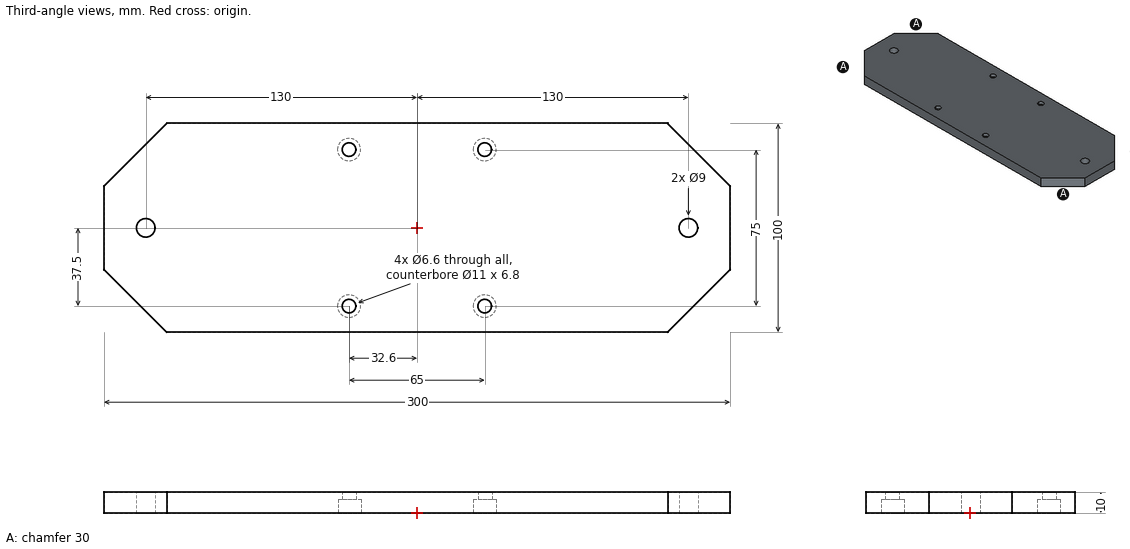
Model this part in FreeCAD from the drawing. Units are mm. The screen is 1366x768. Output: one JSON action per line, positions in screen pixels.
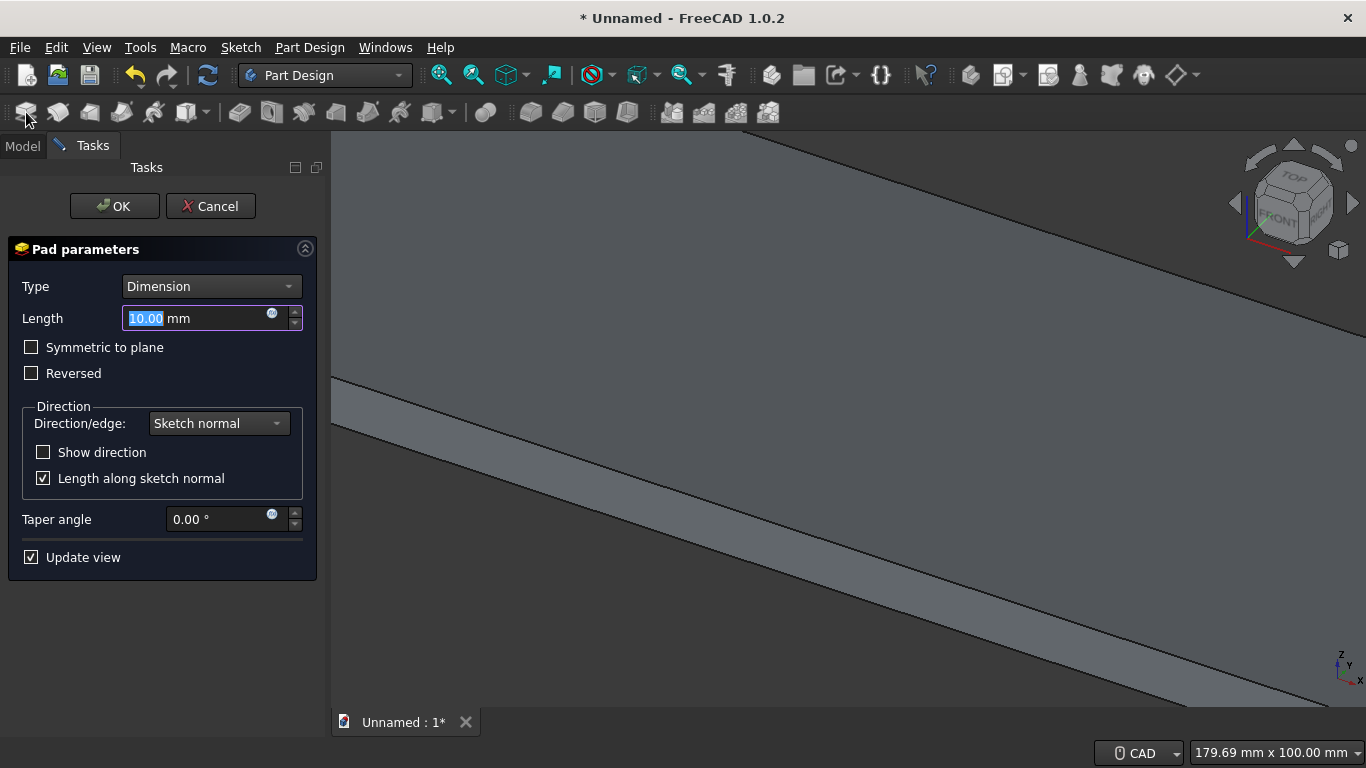
{"action": "type", "text": "10"}
{"action": "key", "text": "Tab"}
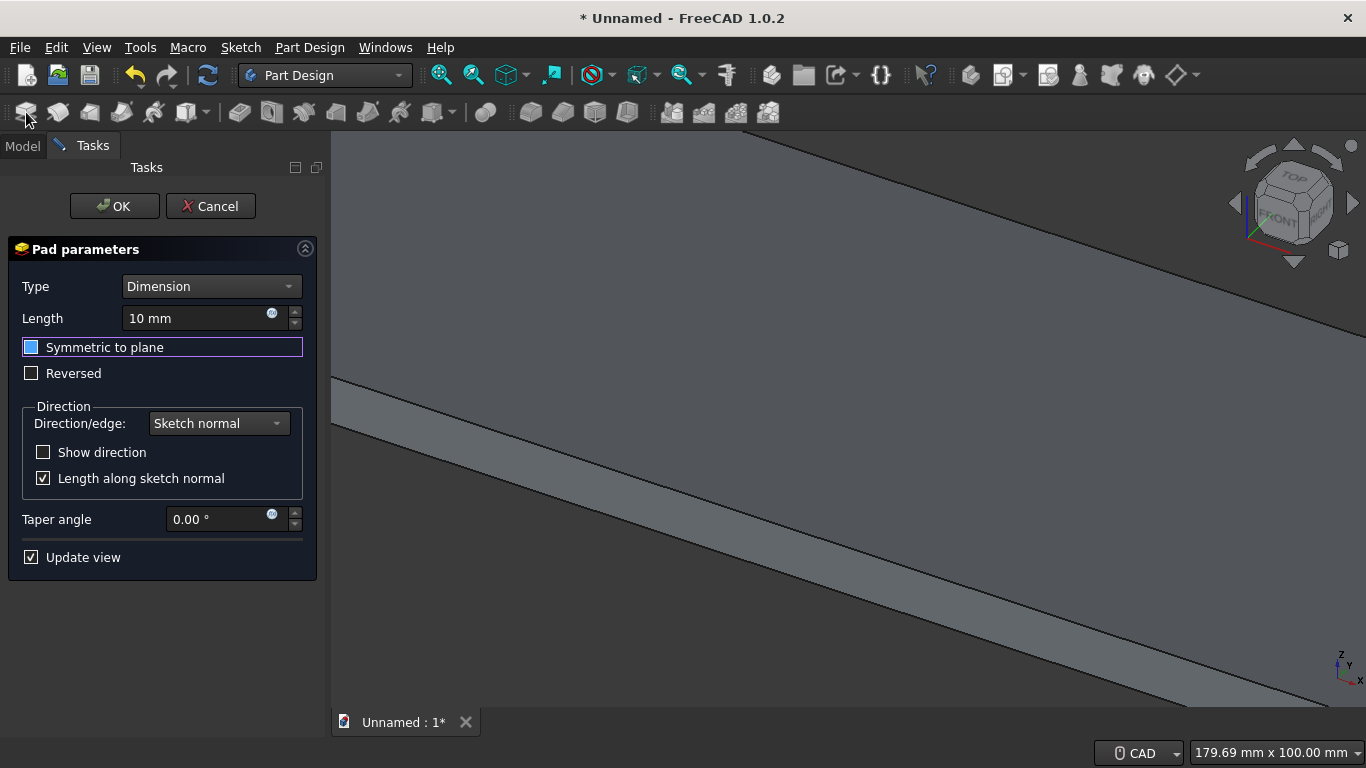
{"action": "left_click", "coordinate": [115, 206]}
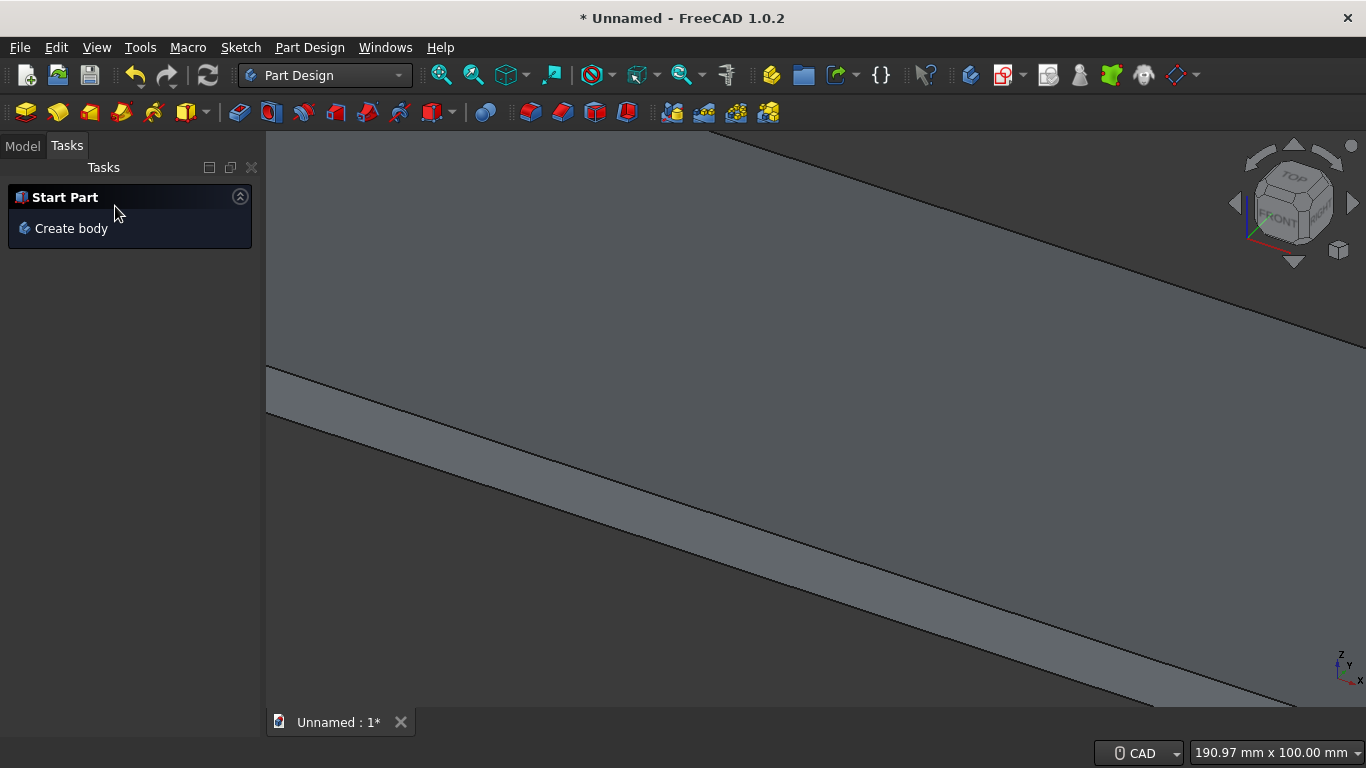
{"action": "key", "text": "v f"}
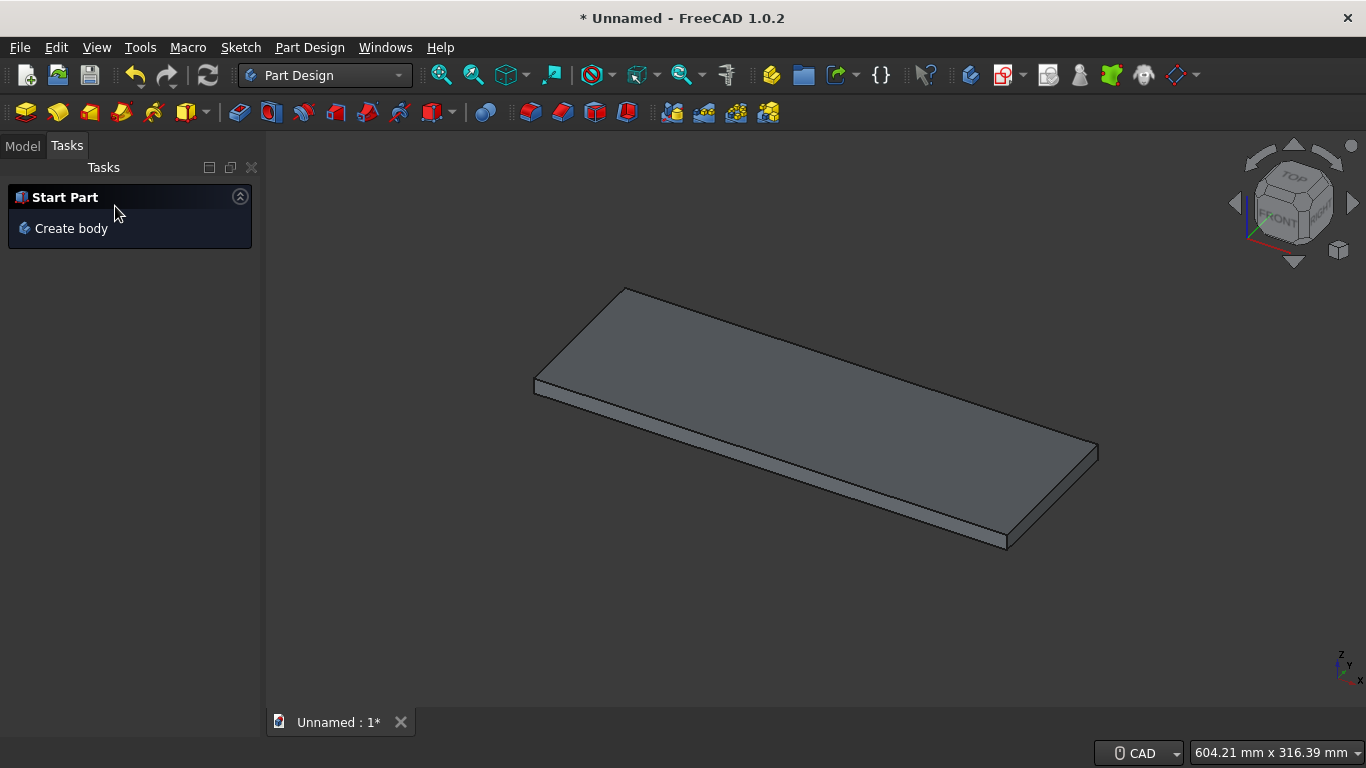
{"action": "key", "text": "5"}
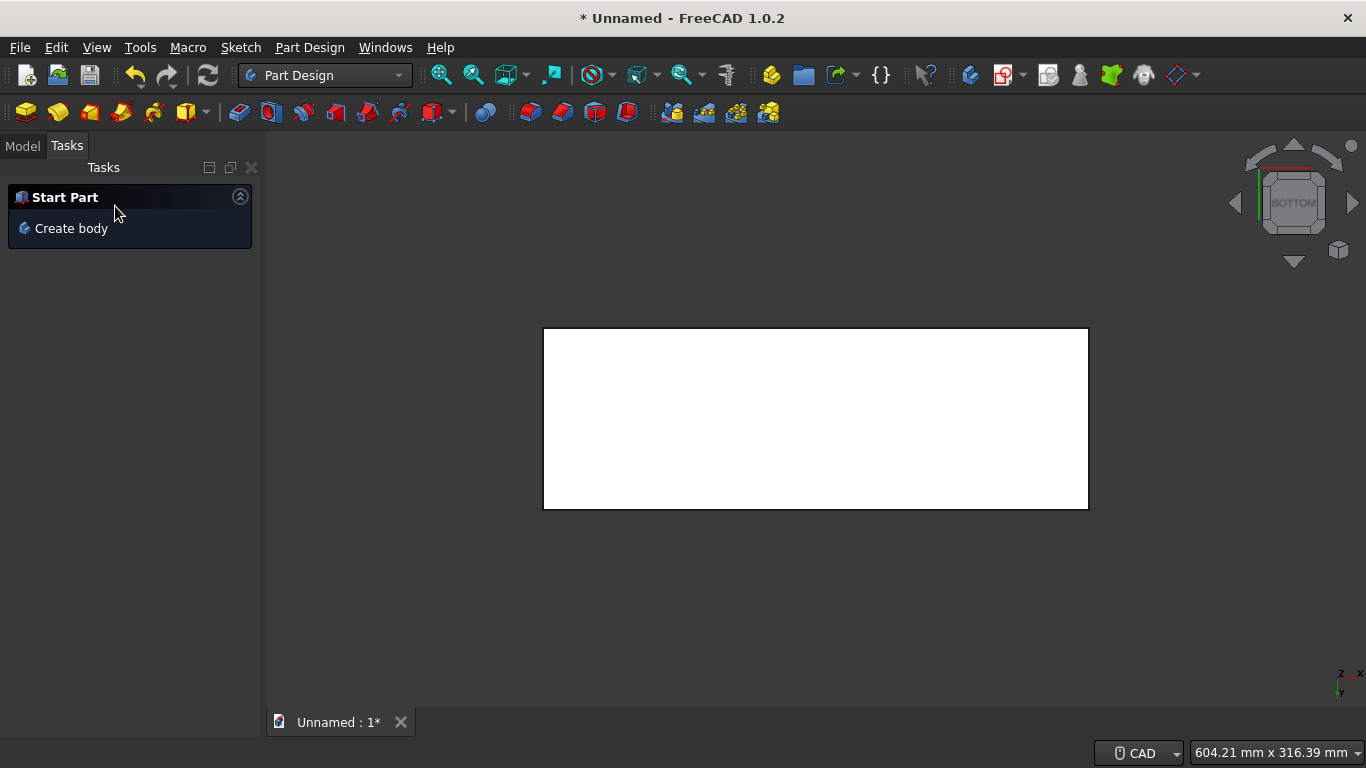
{"action": "left_click", "coordinate": [972, 418]}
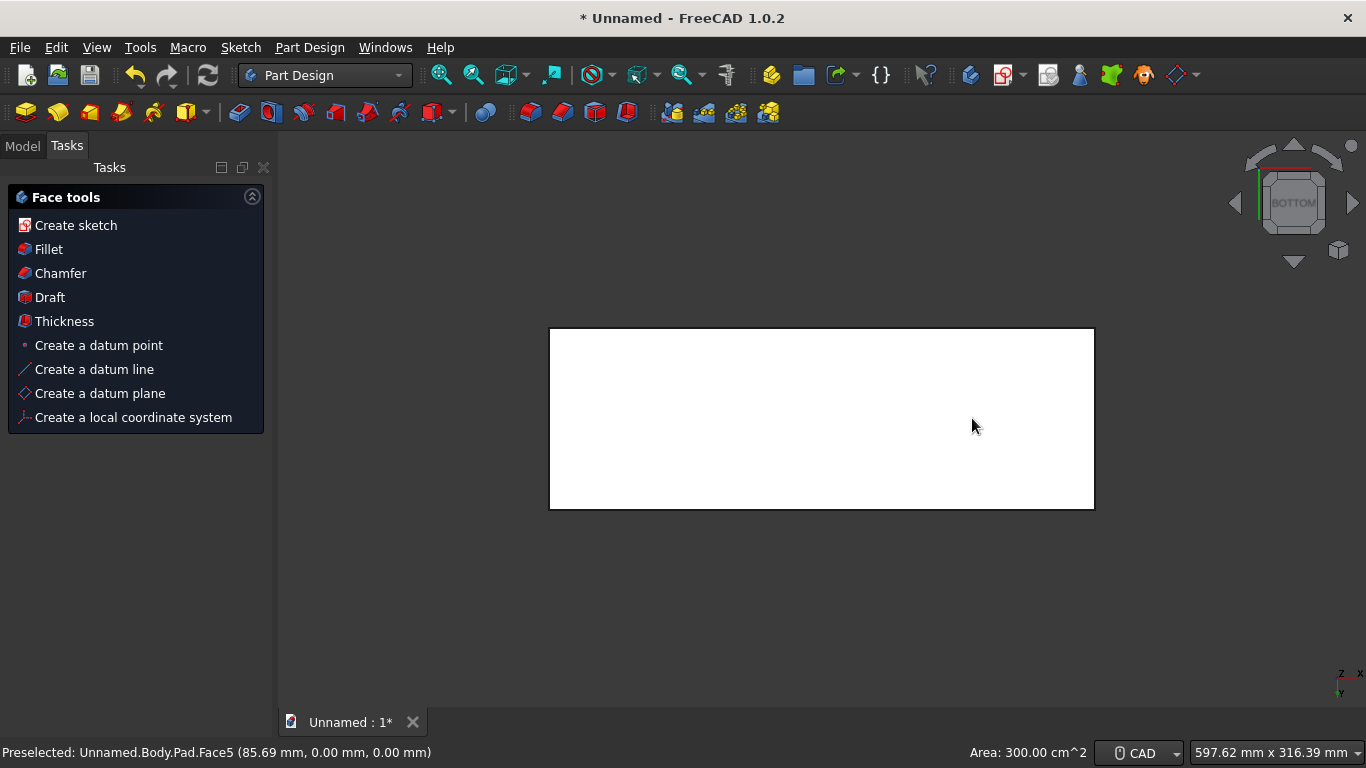
{"action": "left_click", "coordinate": [1004, 76]}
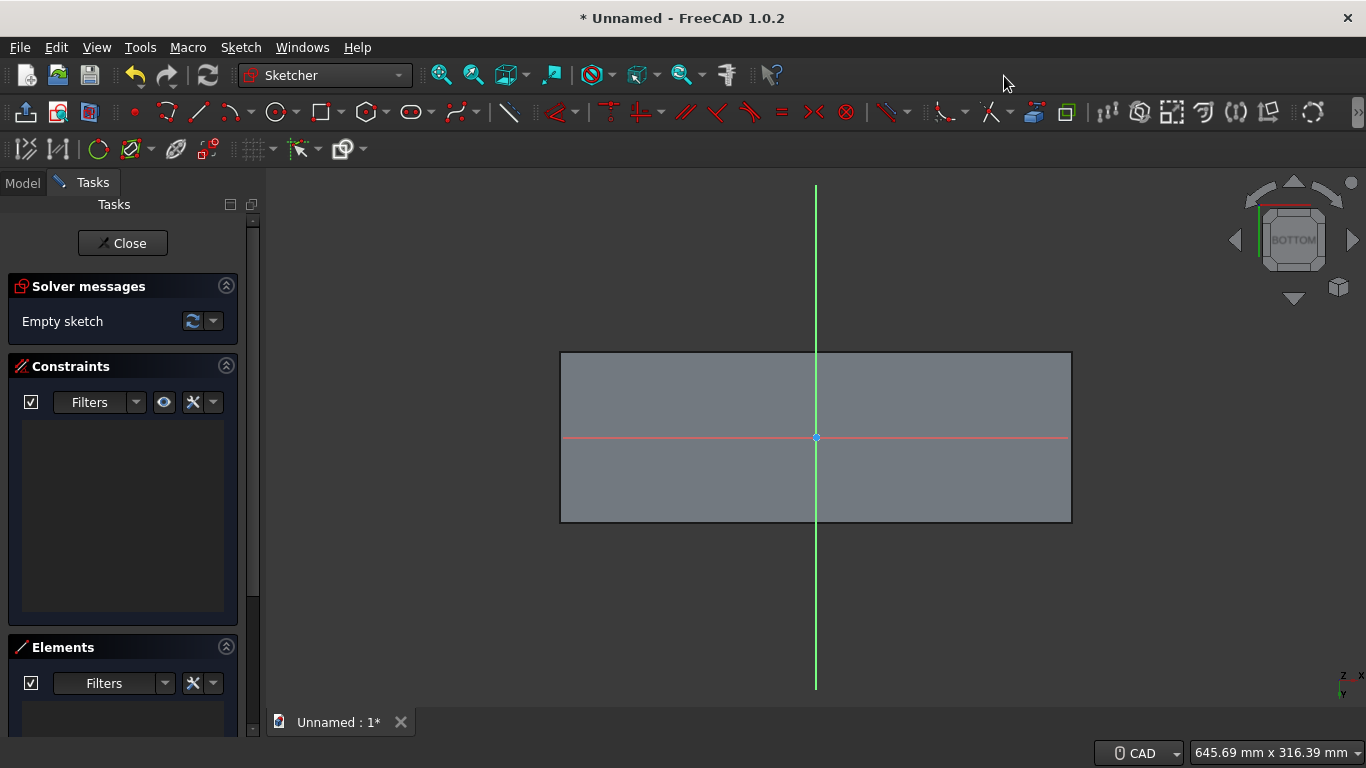
{"action": "scroll", "coordinate": [872, 438], "scroll_direction": "up", "scroll_amount": 4}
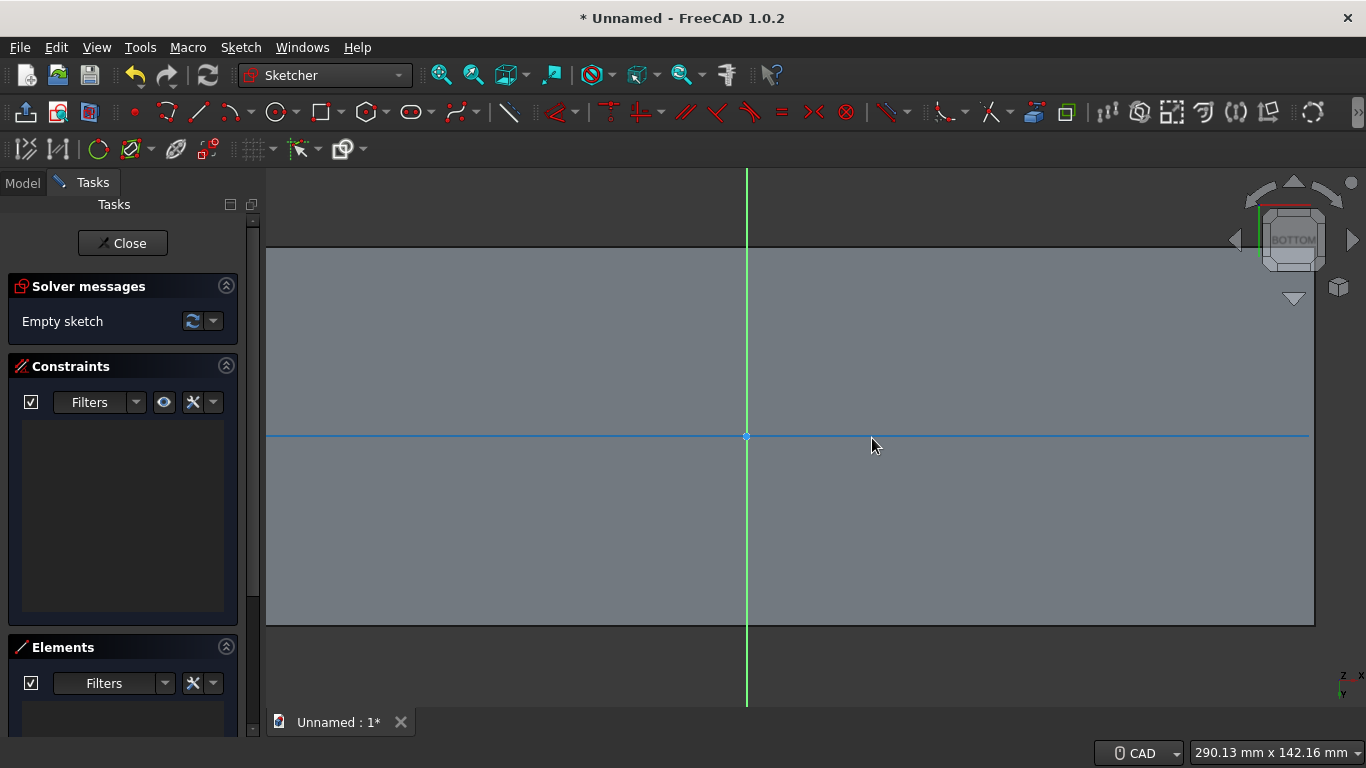
{"action": "key", "text": "g c"}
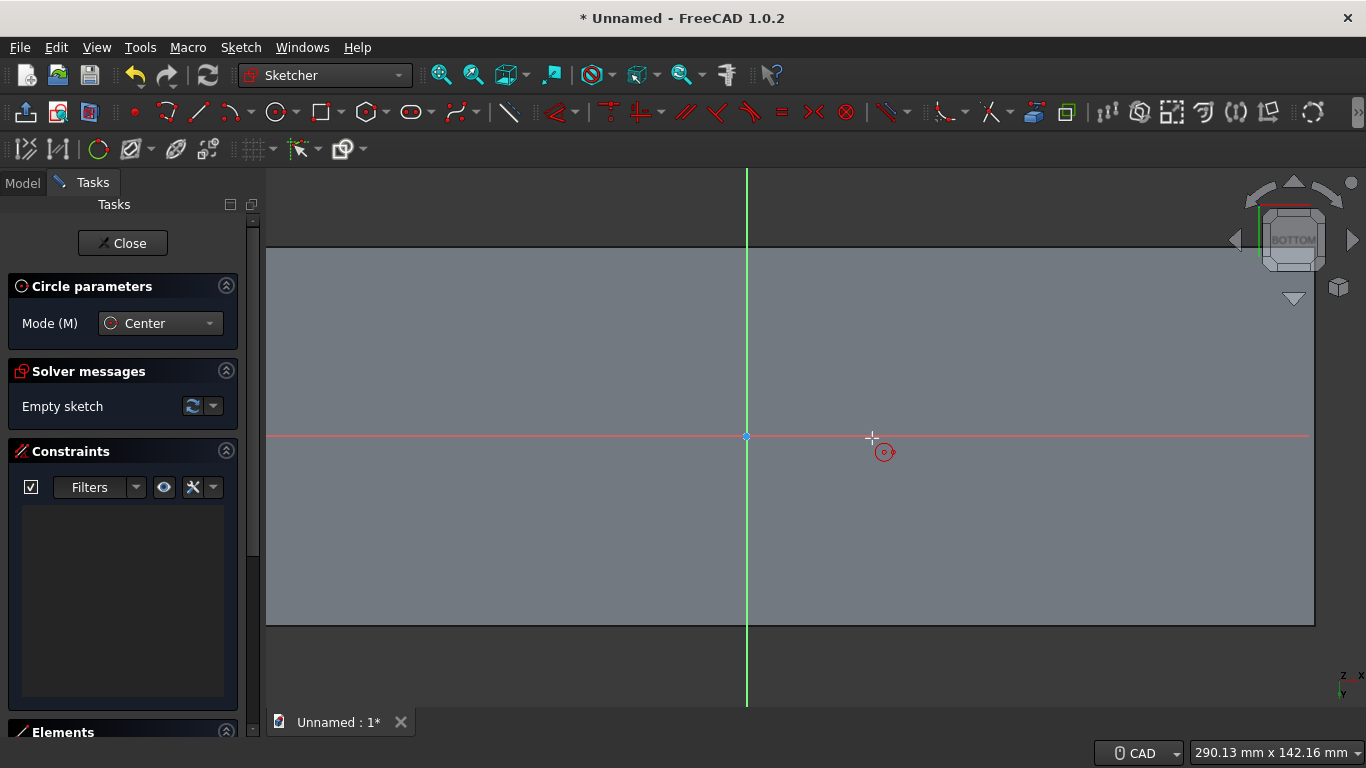
{"action": "scroll", "coordinate": [623, 294], "scroll_direction": "up", "scroll_amount": 3}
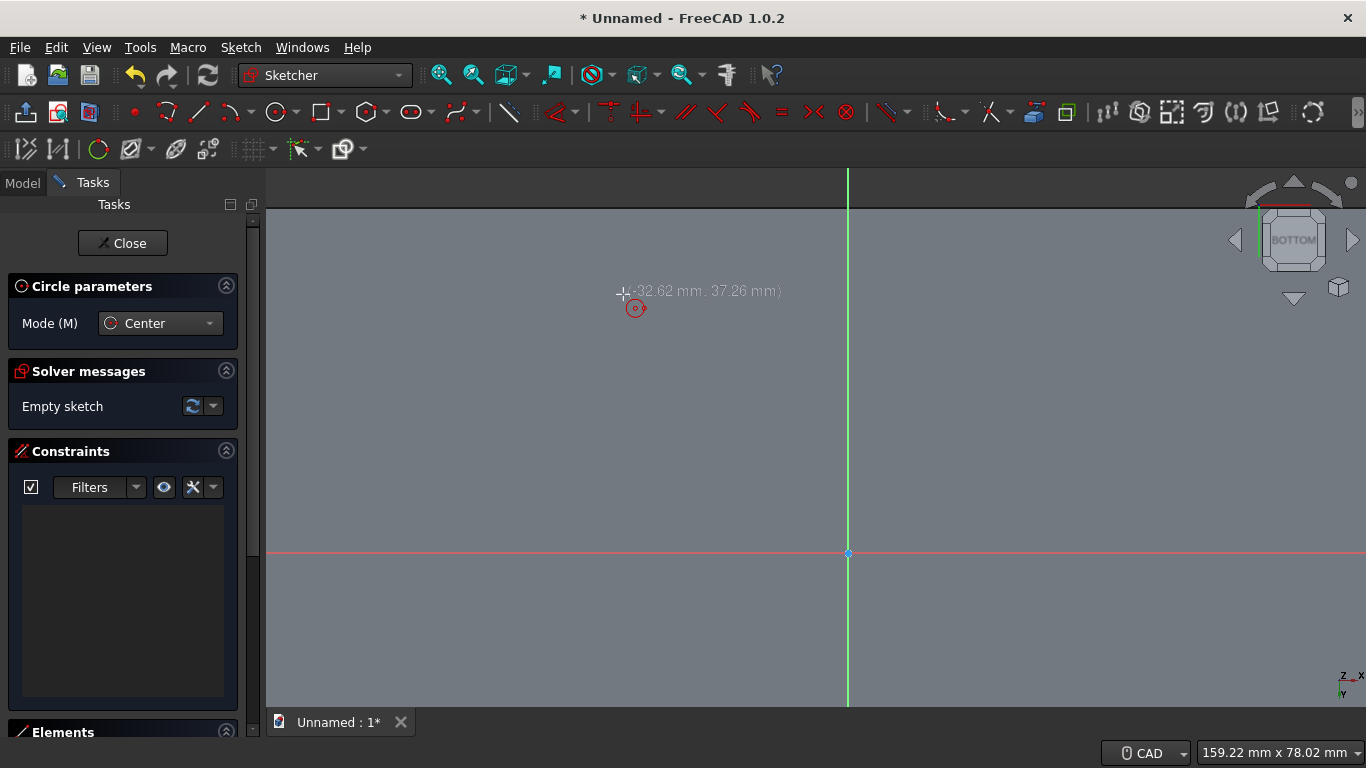
{"action": "left_click", "coordinate": [623, 294]}
{"action": "mouse_move", "coordinate": [639, 278]}